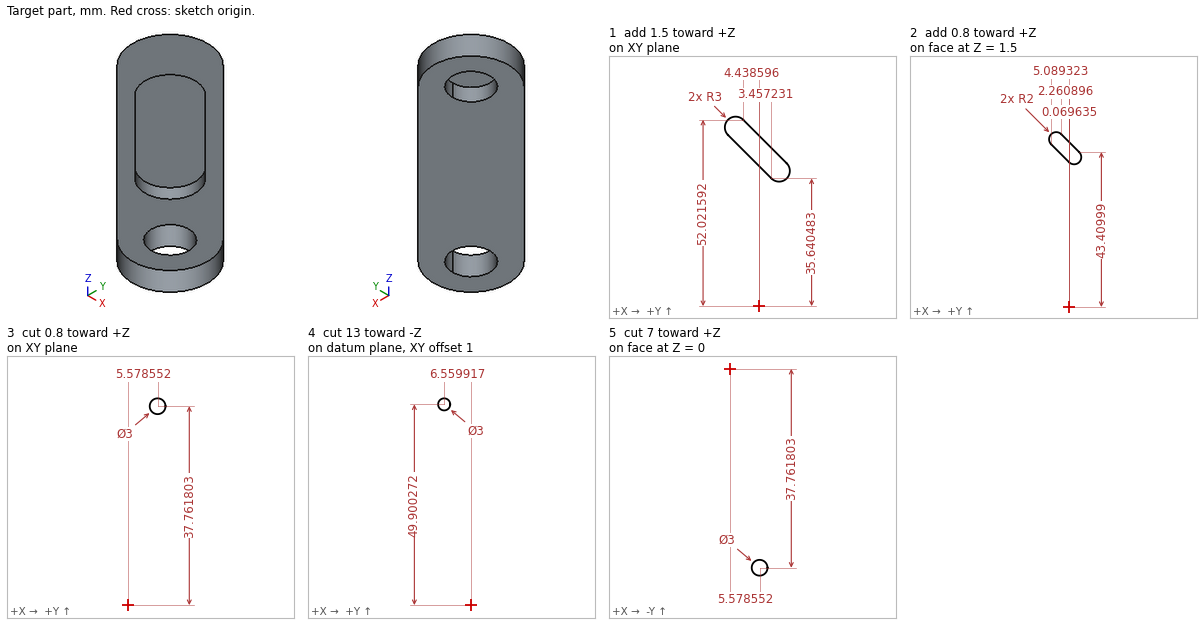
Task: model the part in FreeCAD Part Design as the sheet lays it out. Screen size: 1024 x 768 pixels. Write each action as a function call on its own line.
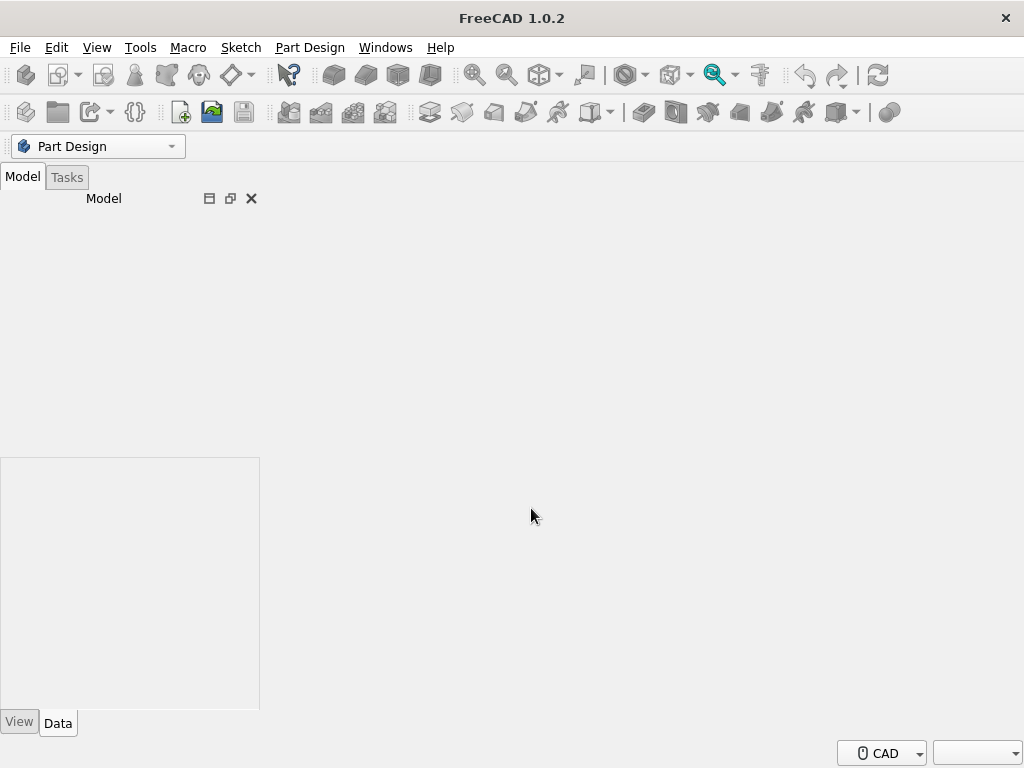
click(180, 112)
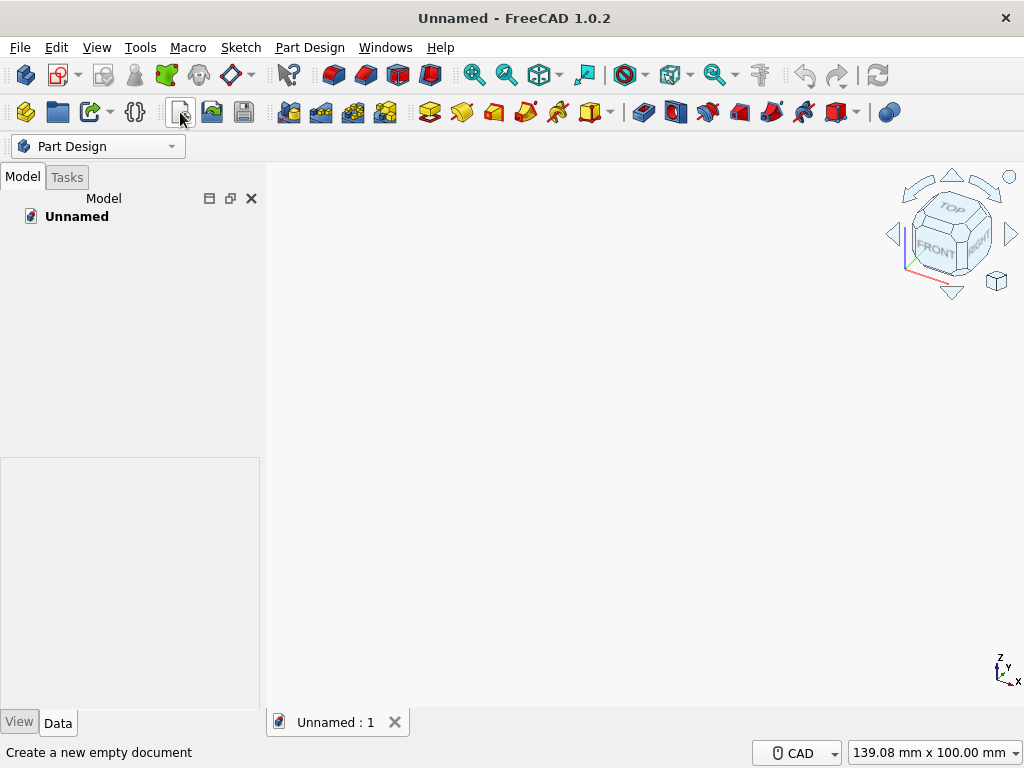
click(58, 76)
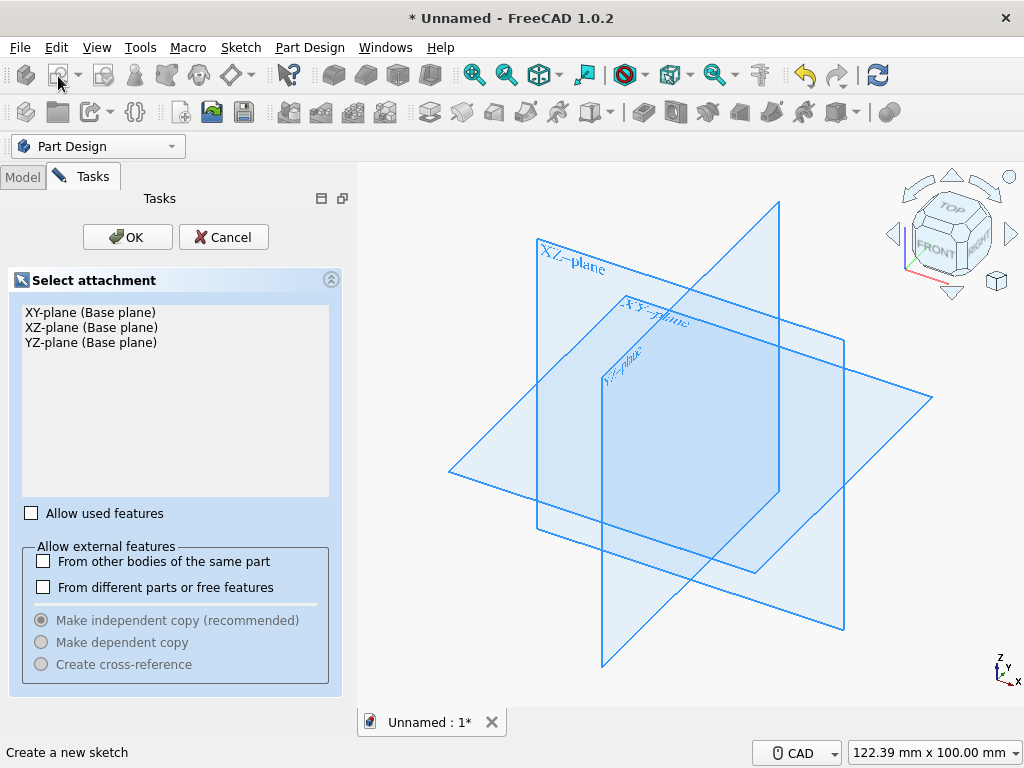
click(82, 312)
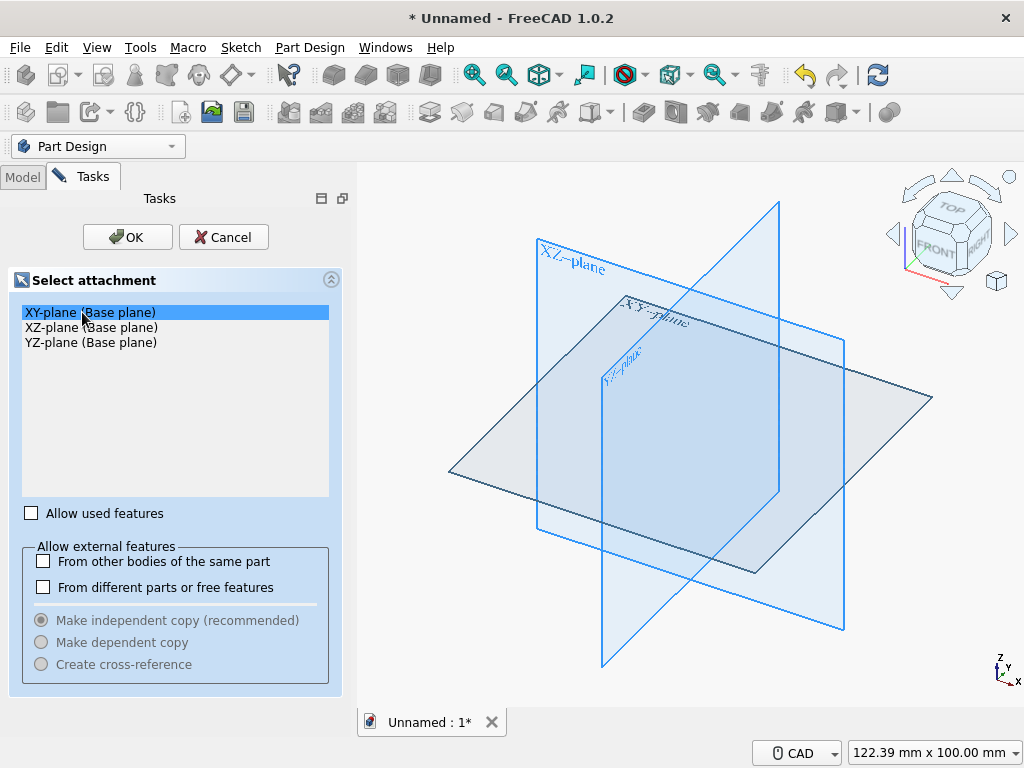
click(128, 237)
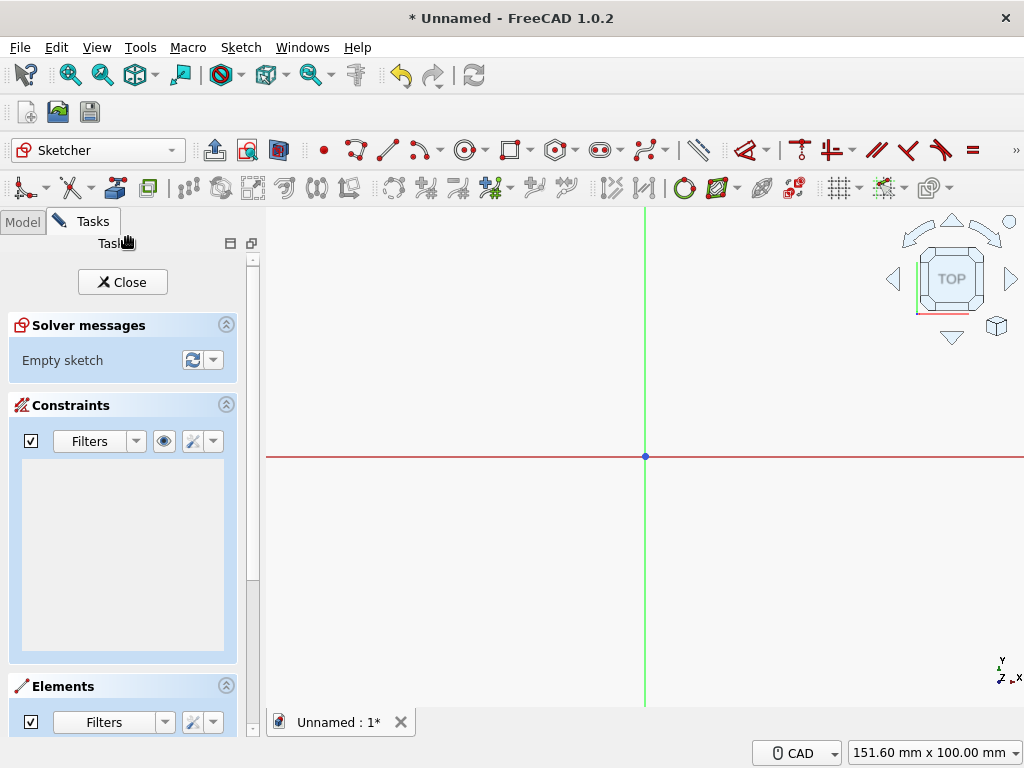
scroll(576, 457, down, 5)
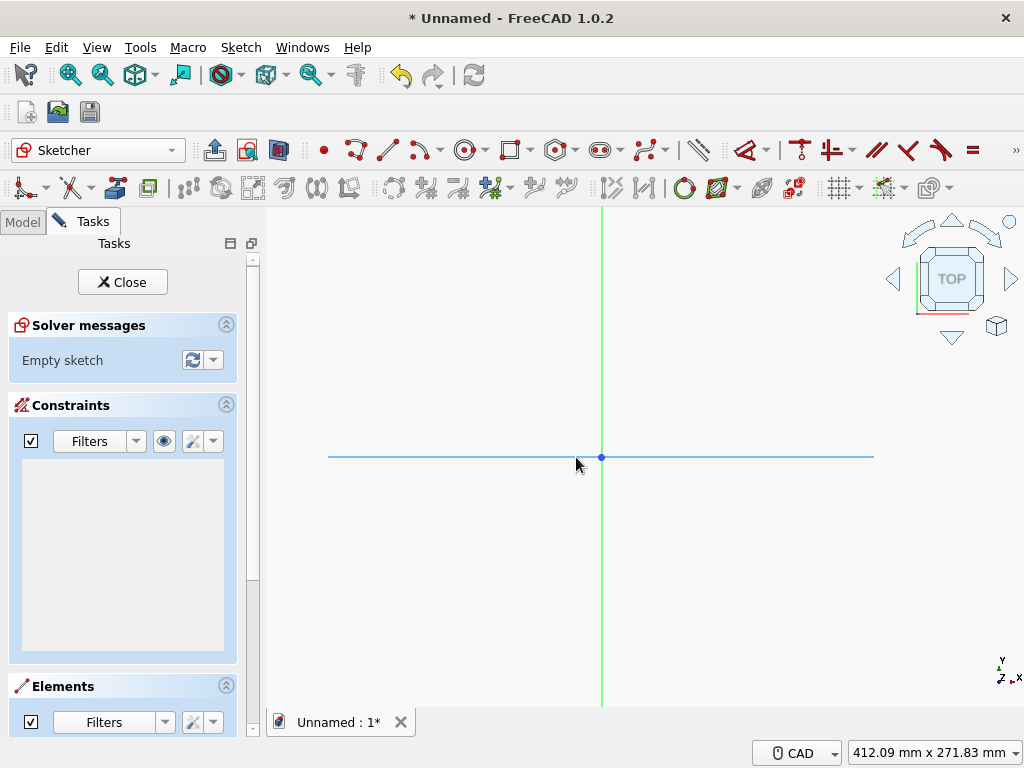
scroll(603, 369, up, 12)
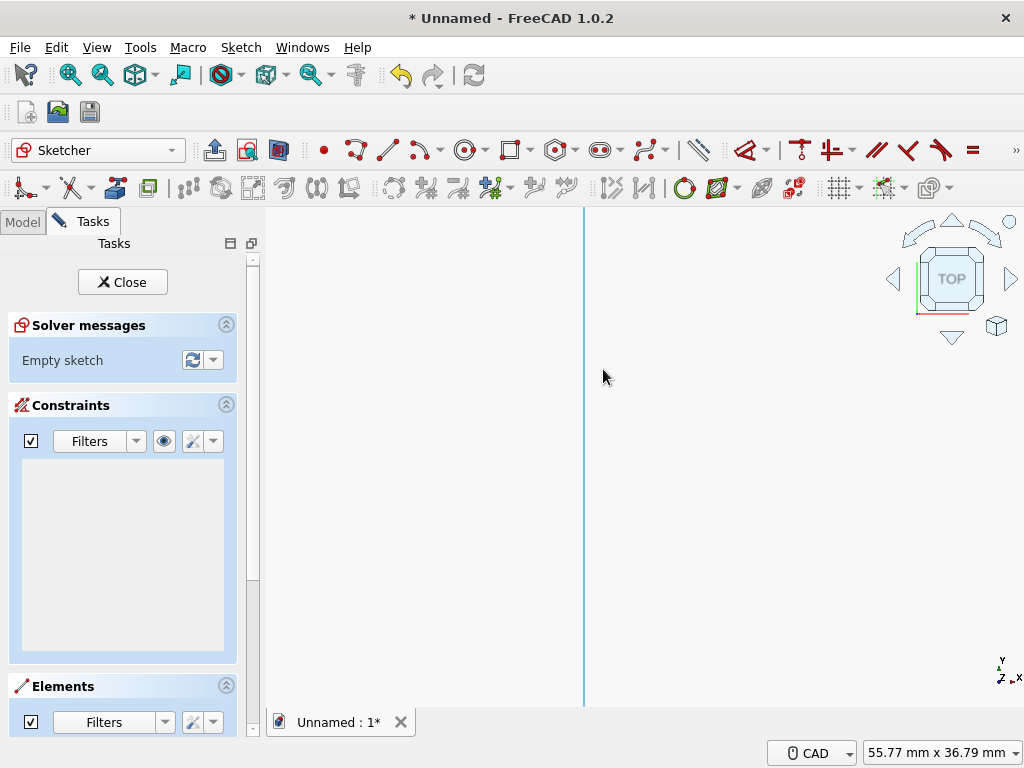
key(g)
key(s)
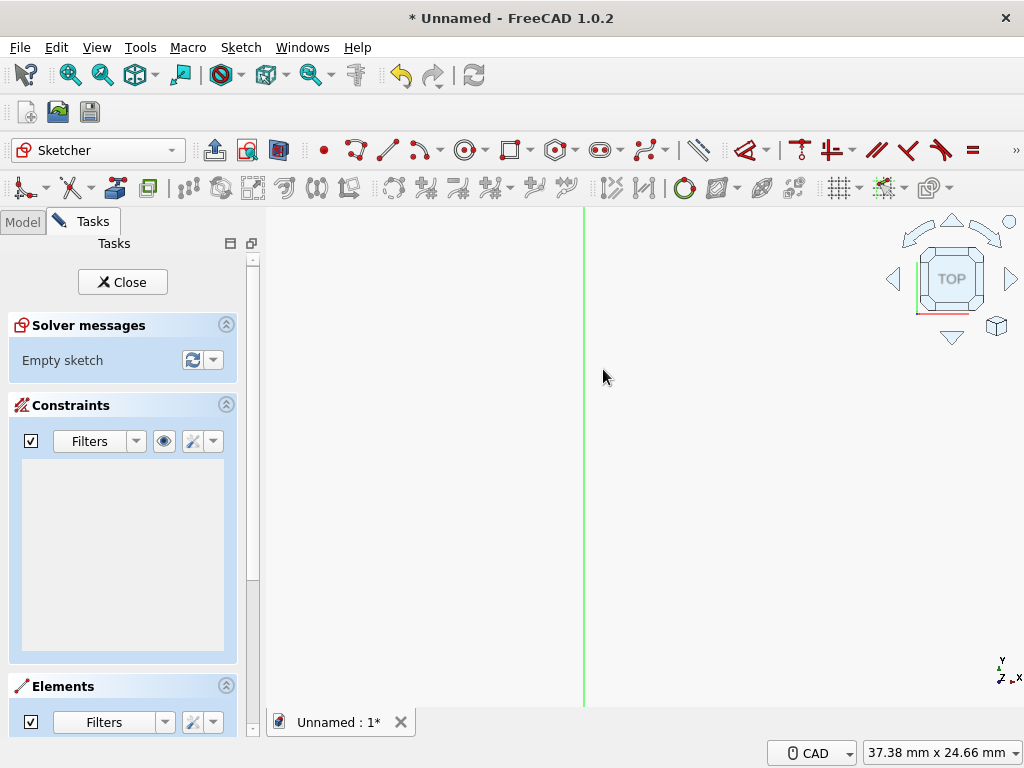
click(451, 327)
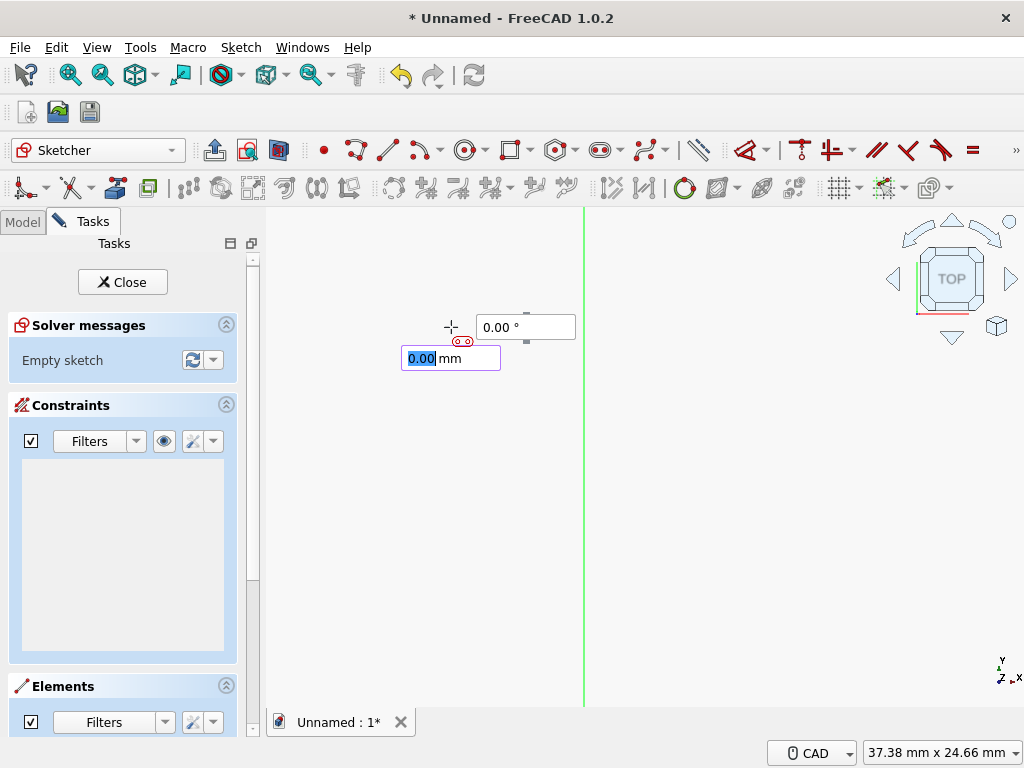
click(697, 574)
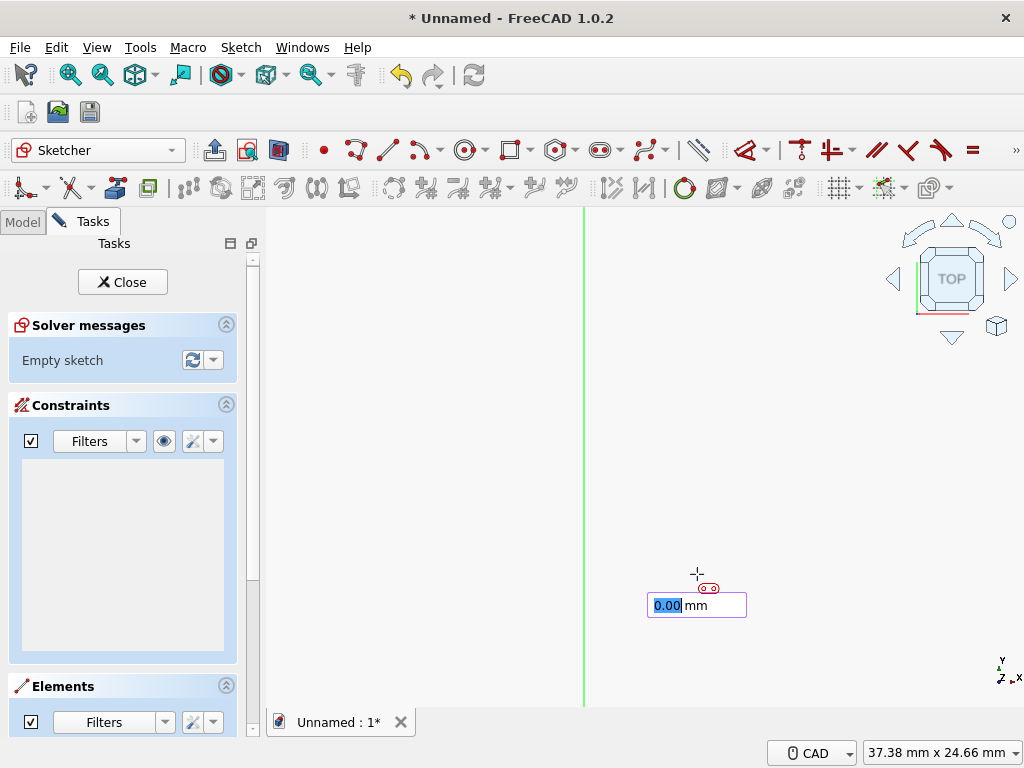
click(617, 408)
key(Escape)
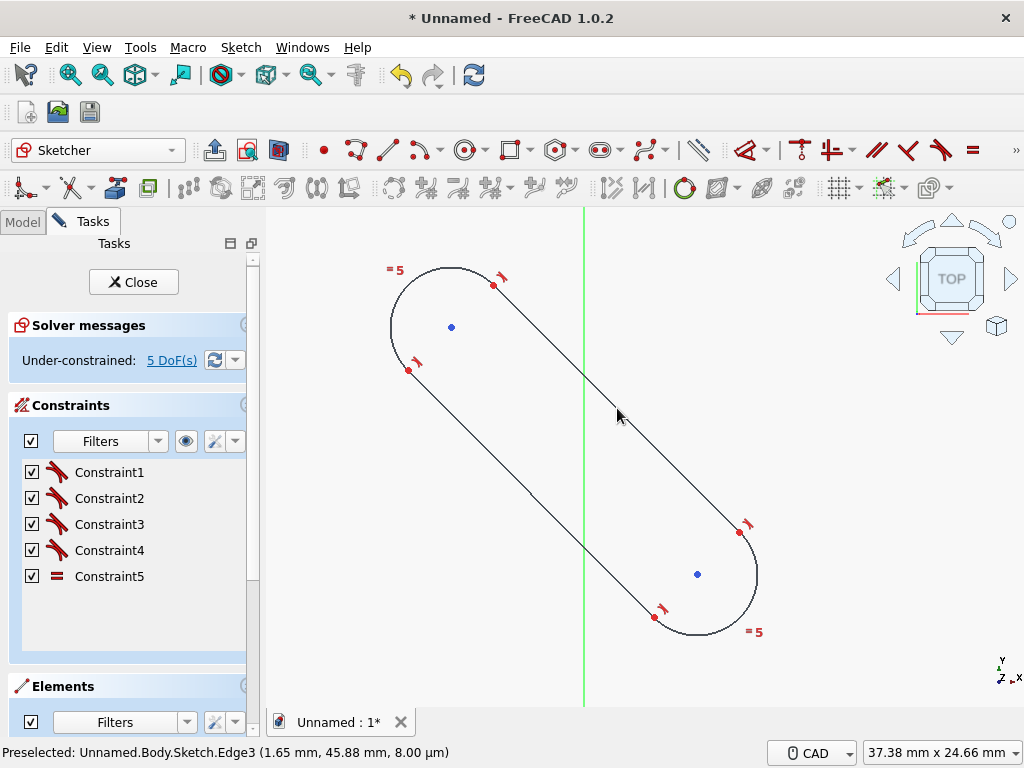
click(746, 150)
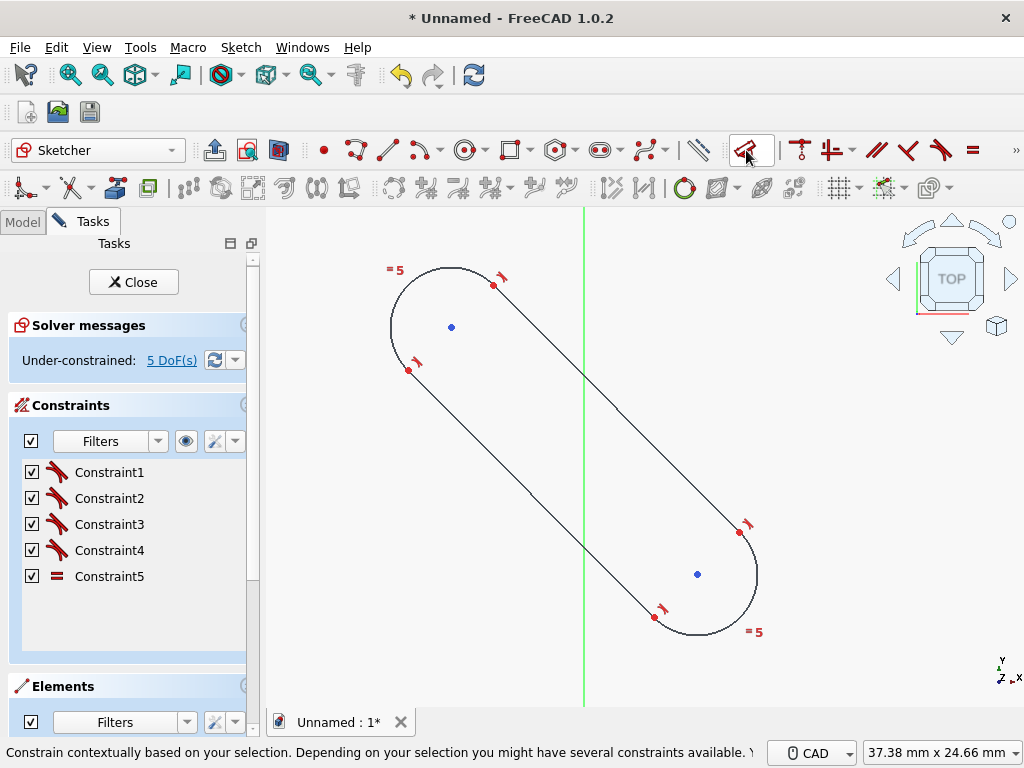
click(442, 268)
click(437, 236)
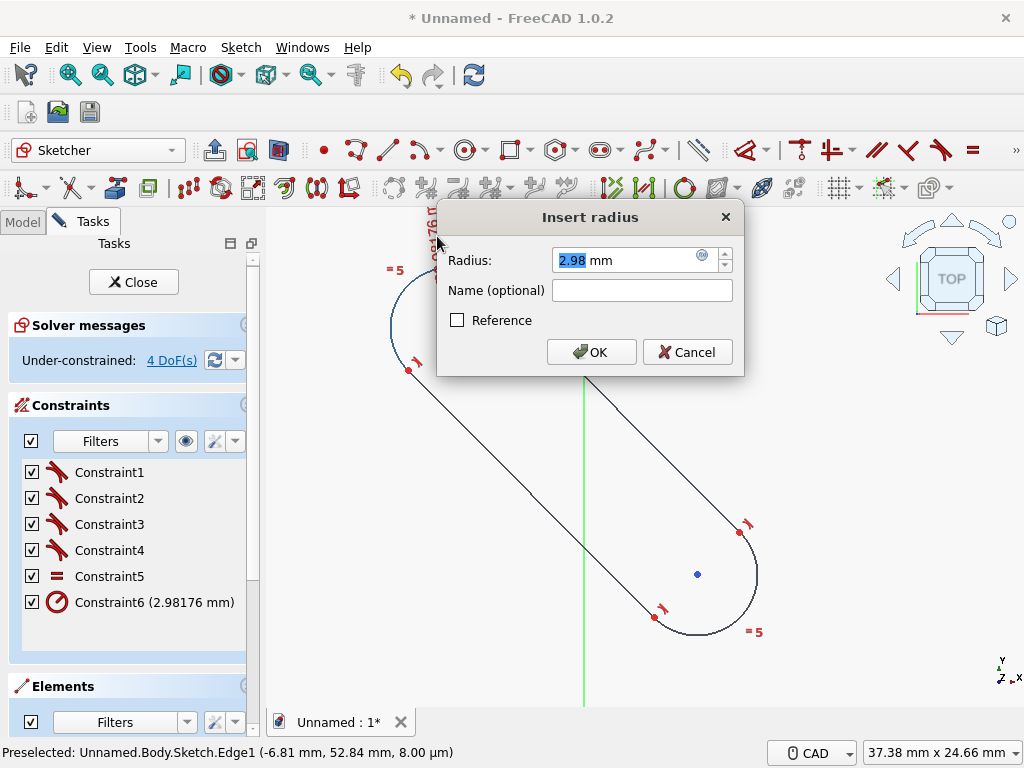
text(3)
key(Return)